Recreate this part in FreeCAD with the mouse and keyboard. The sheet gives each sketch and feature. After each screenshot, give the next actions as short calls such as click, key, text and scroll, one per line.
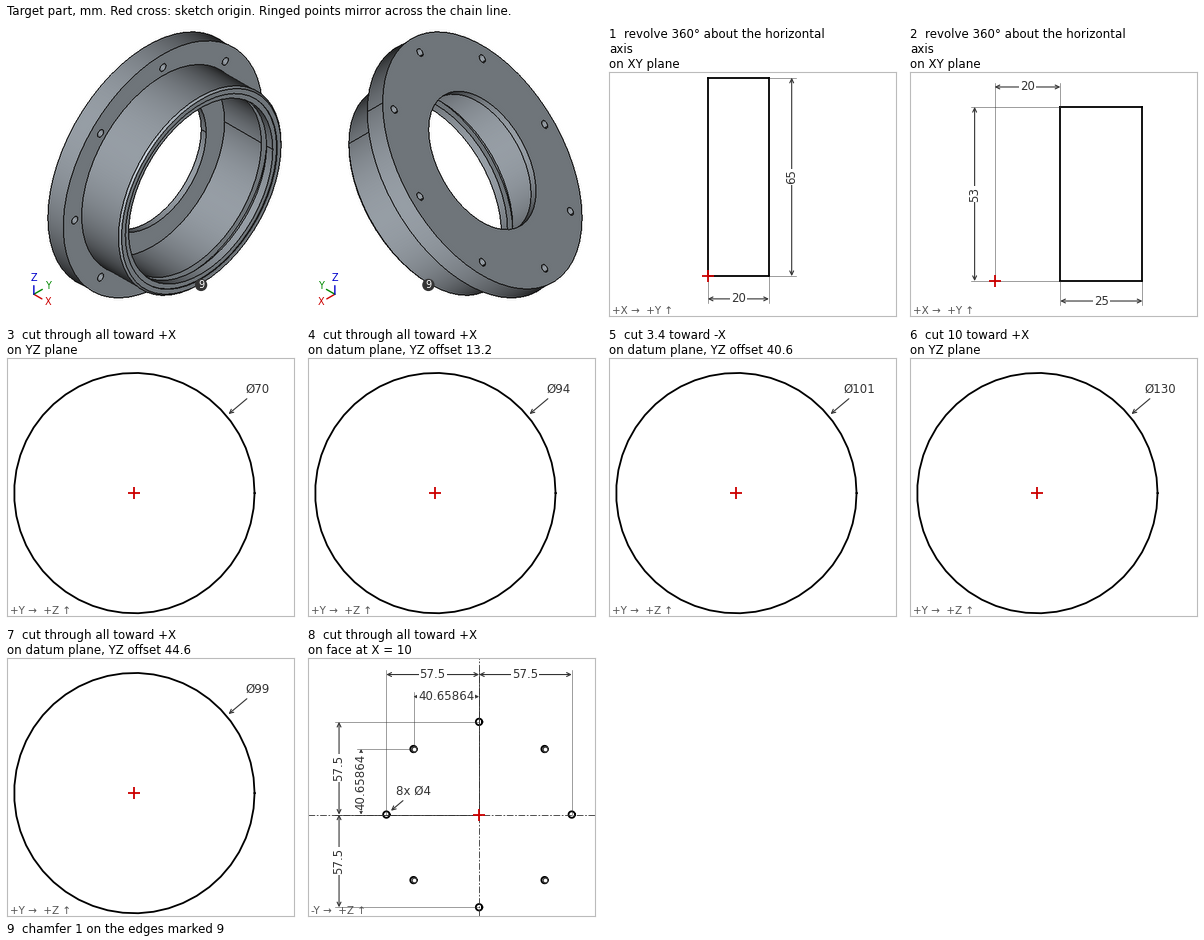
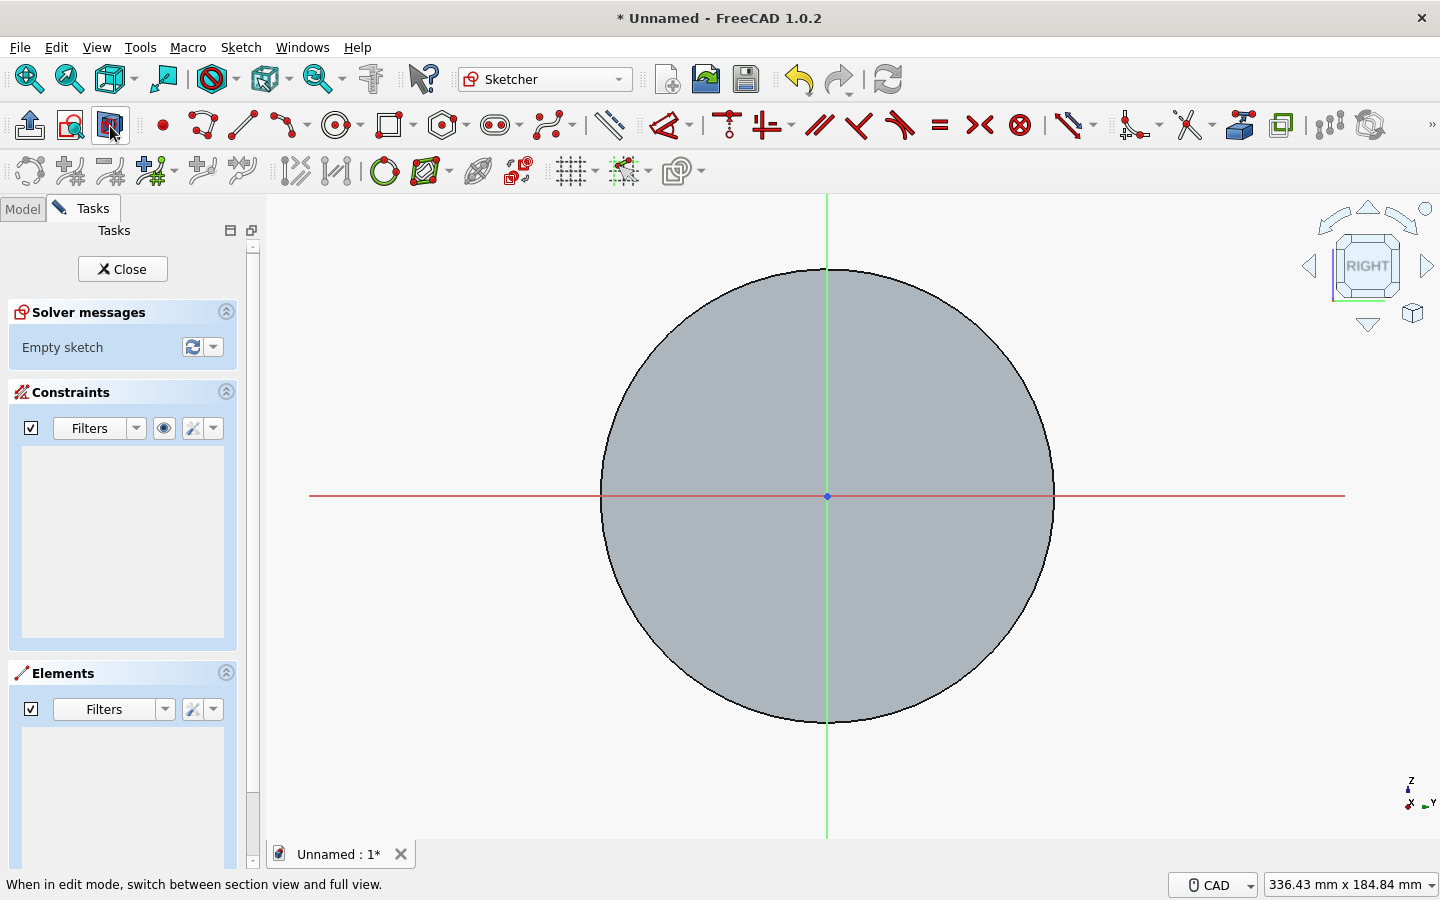
scroll(880, 471, up, 3)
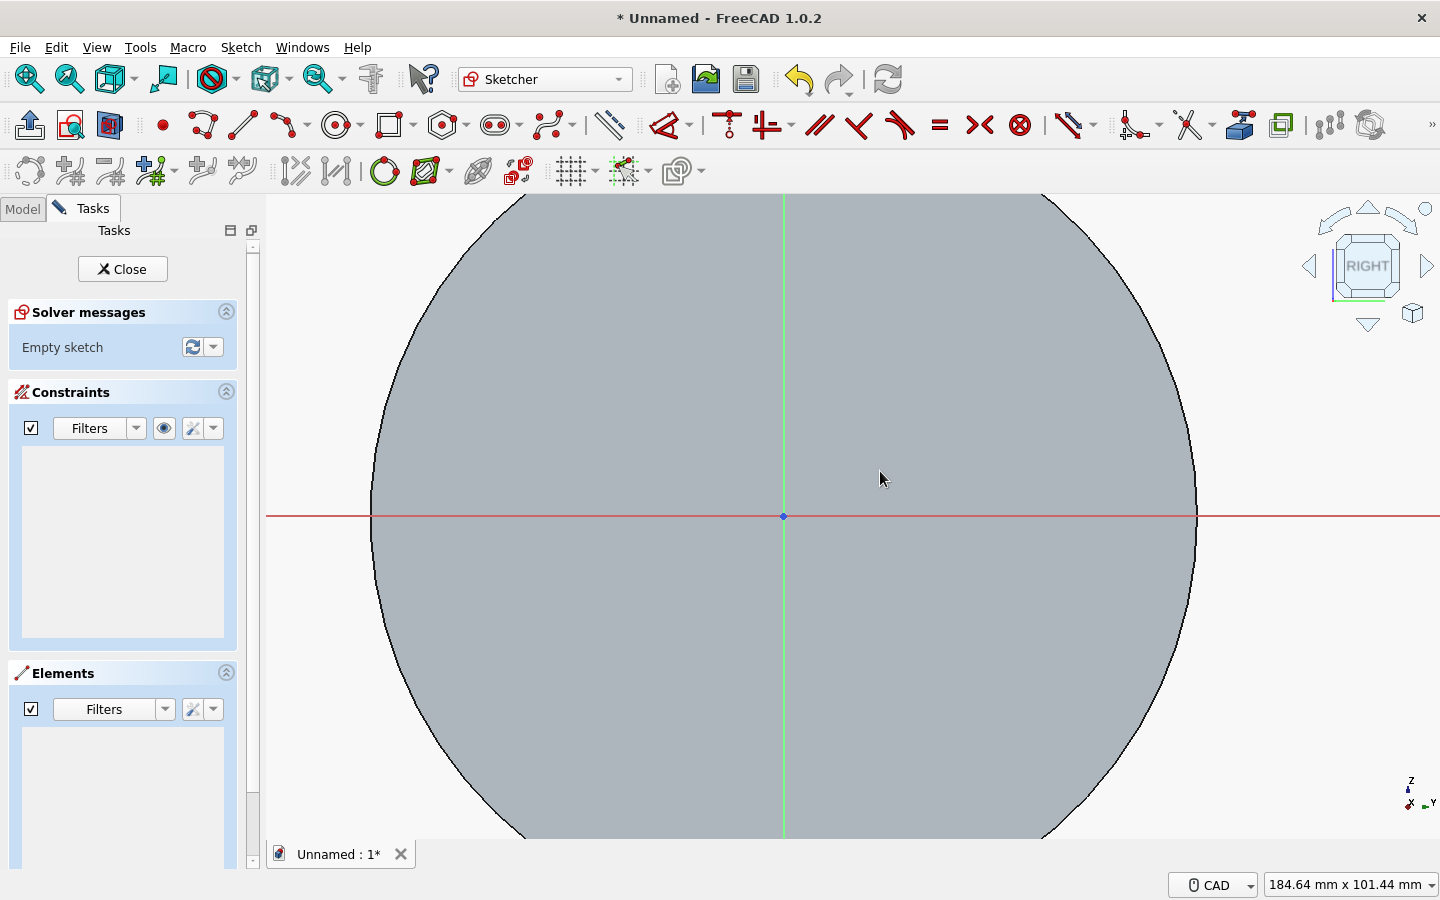
click(336, 126)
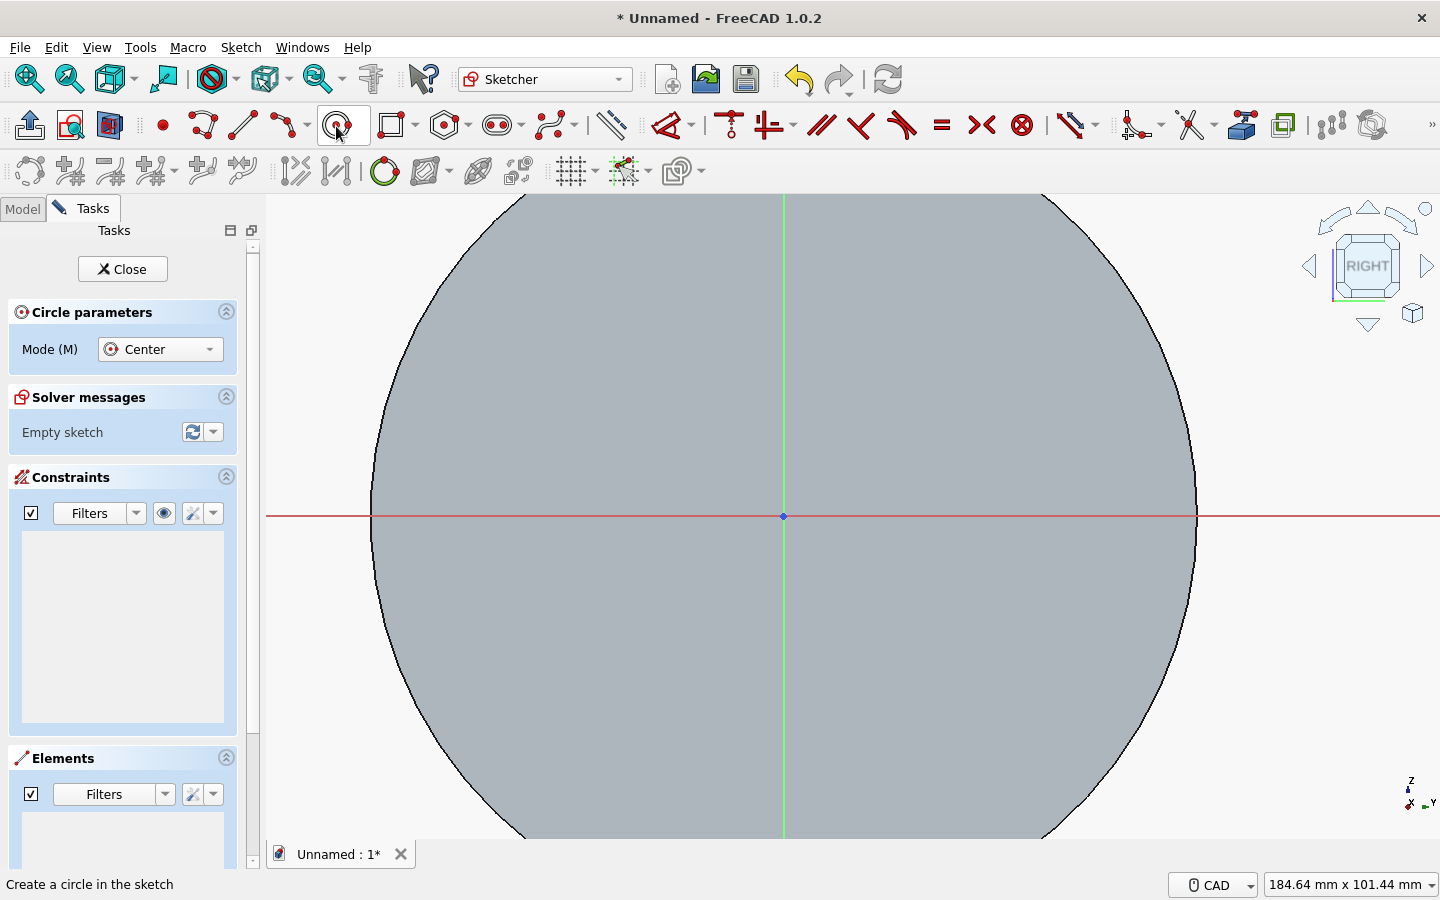
click(784, 516)
click(941, 359)
key(Escape)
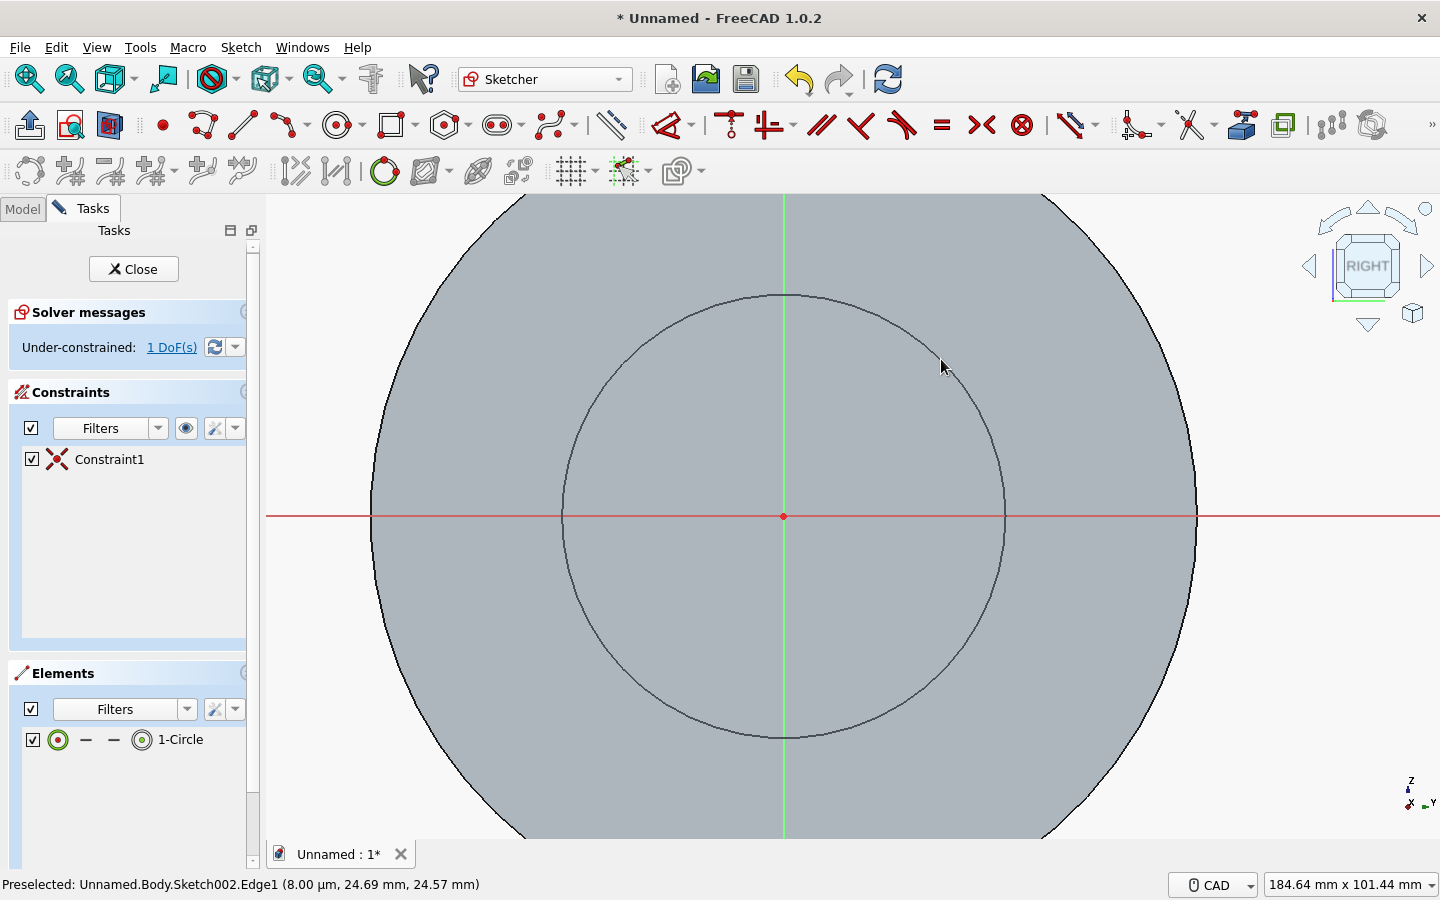
click(666, 126)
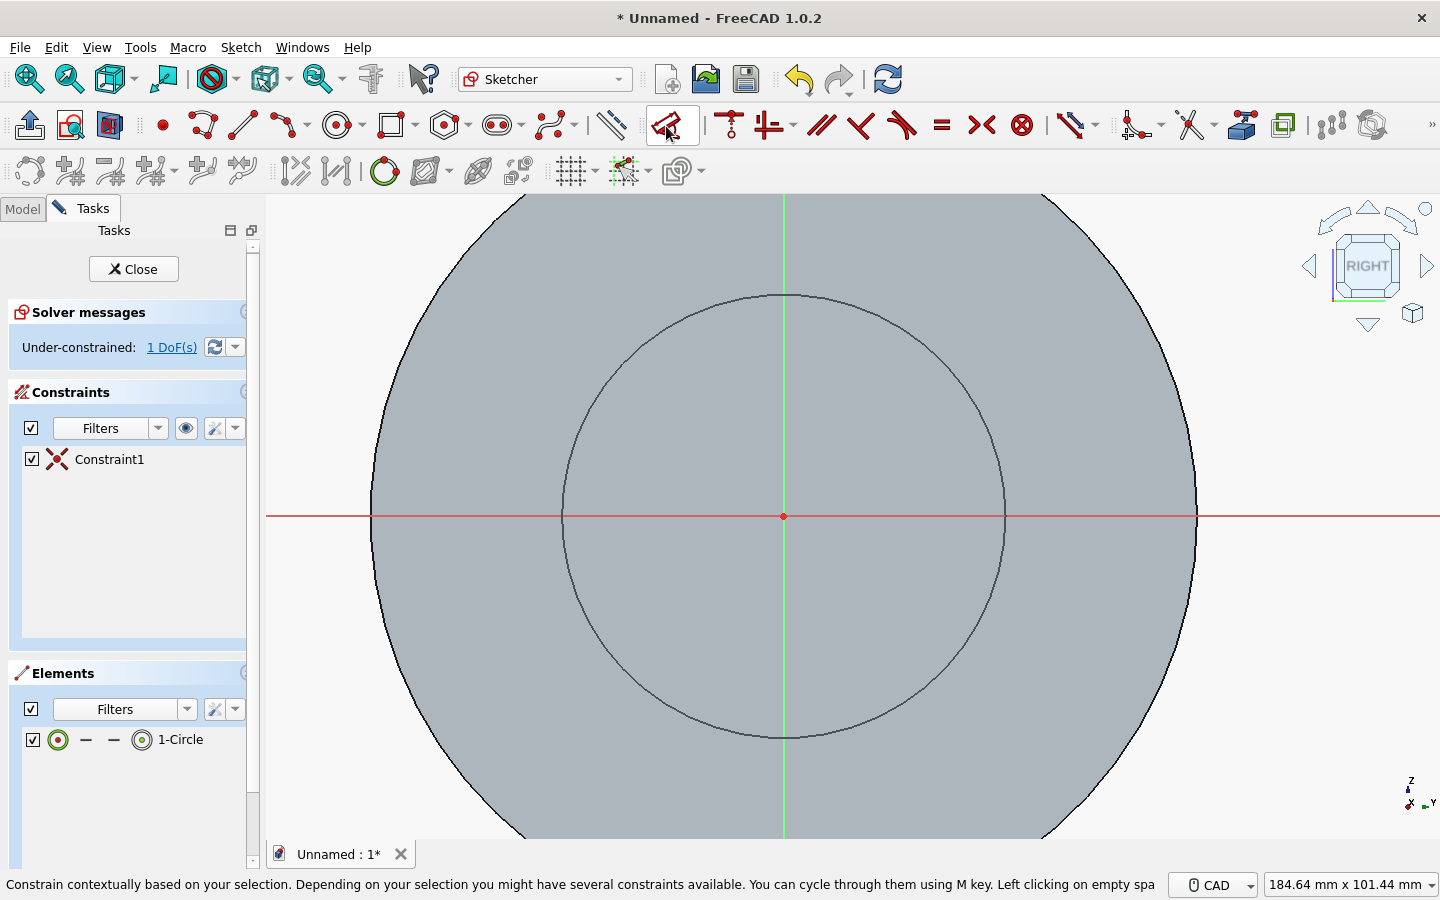
click(940, 359)
click(963, 336)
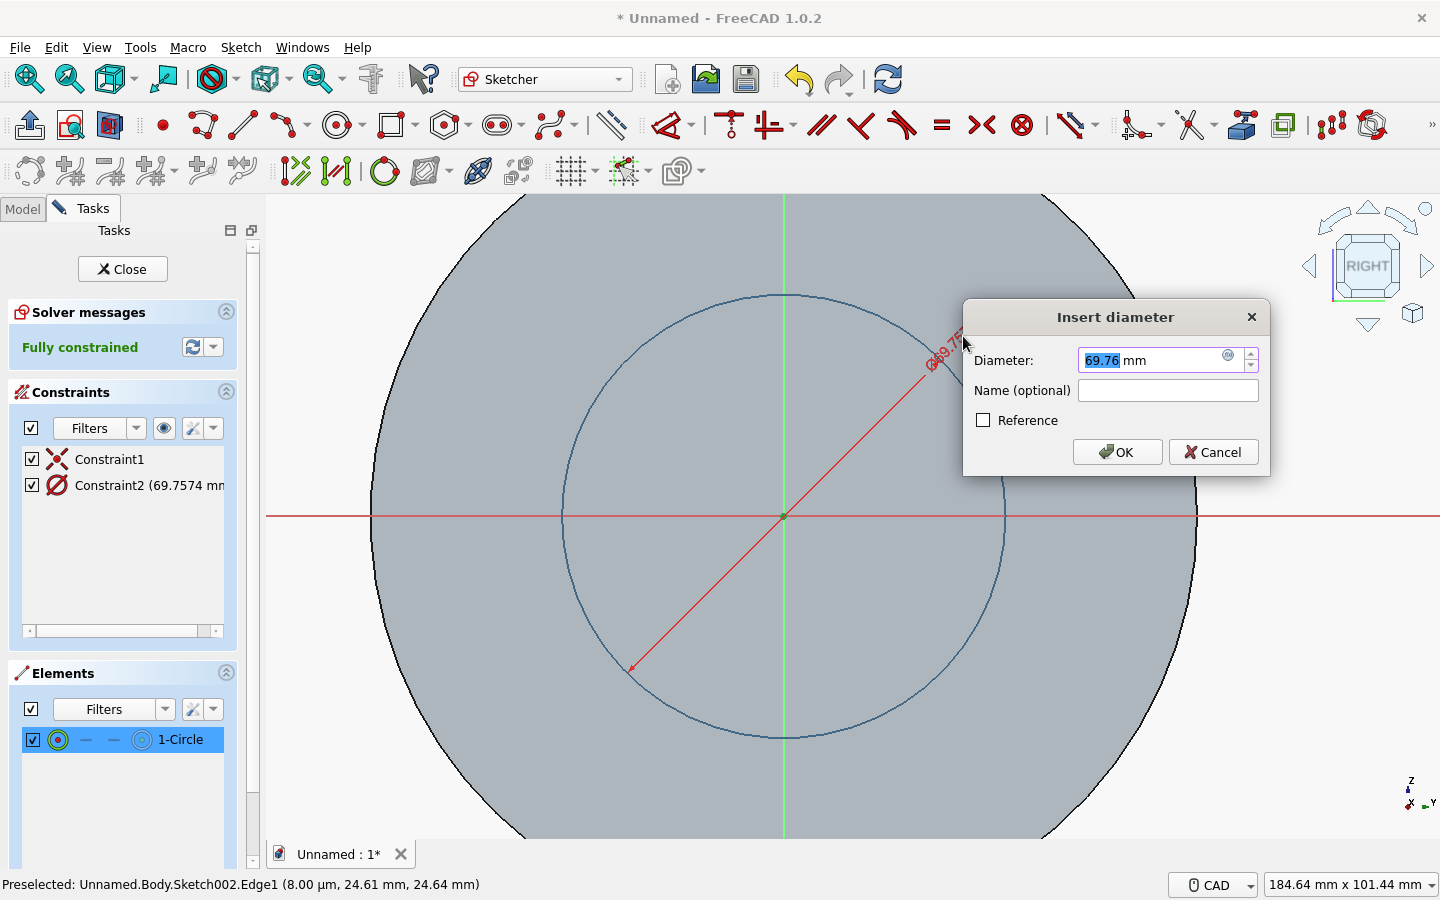
text(70)
key(Return)
key(Escape)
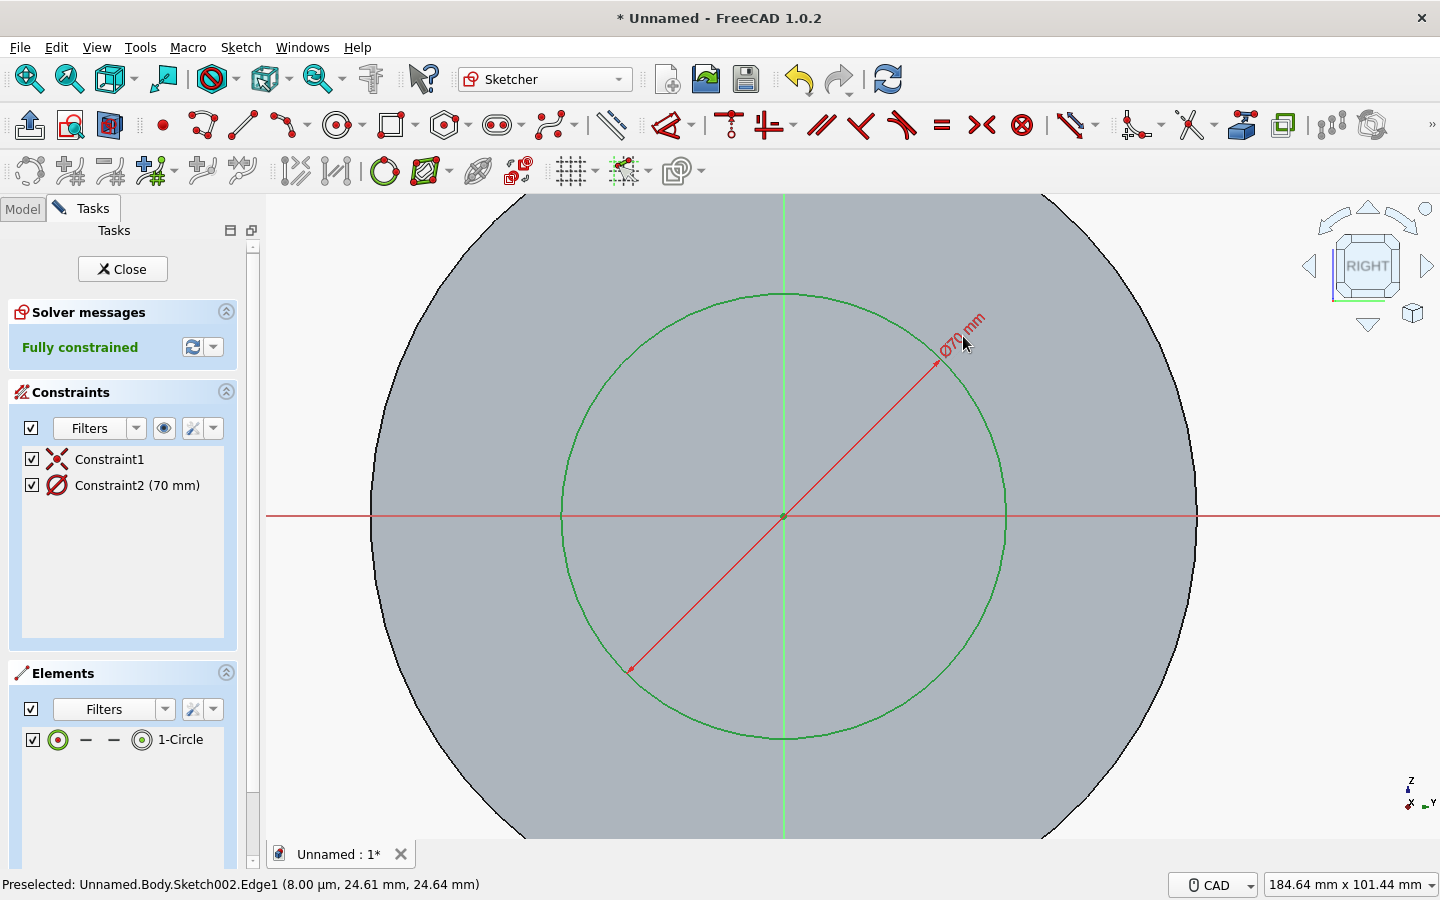
click(123, 269)